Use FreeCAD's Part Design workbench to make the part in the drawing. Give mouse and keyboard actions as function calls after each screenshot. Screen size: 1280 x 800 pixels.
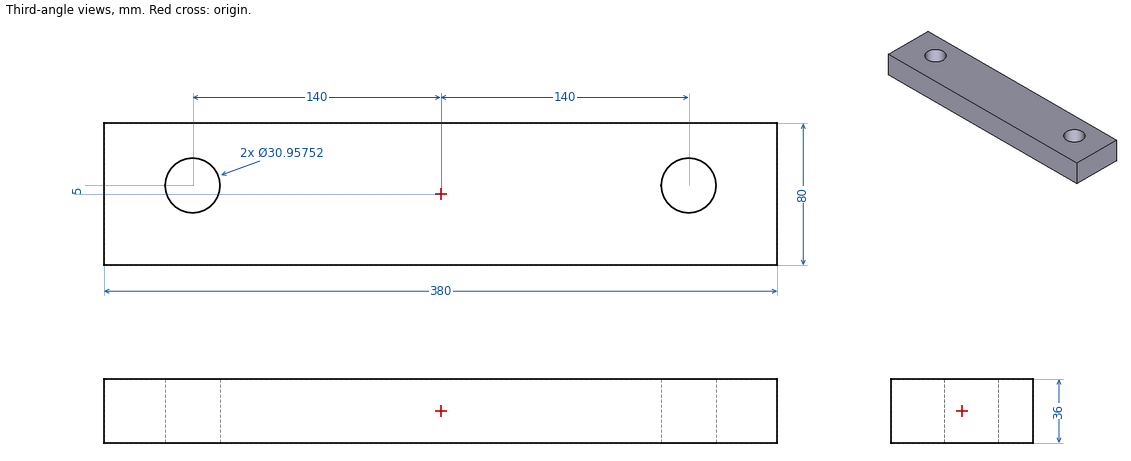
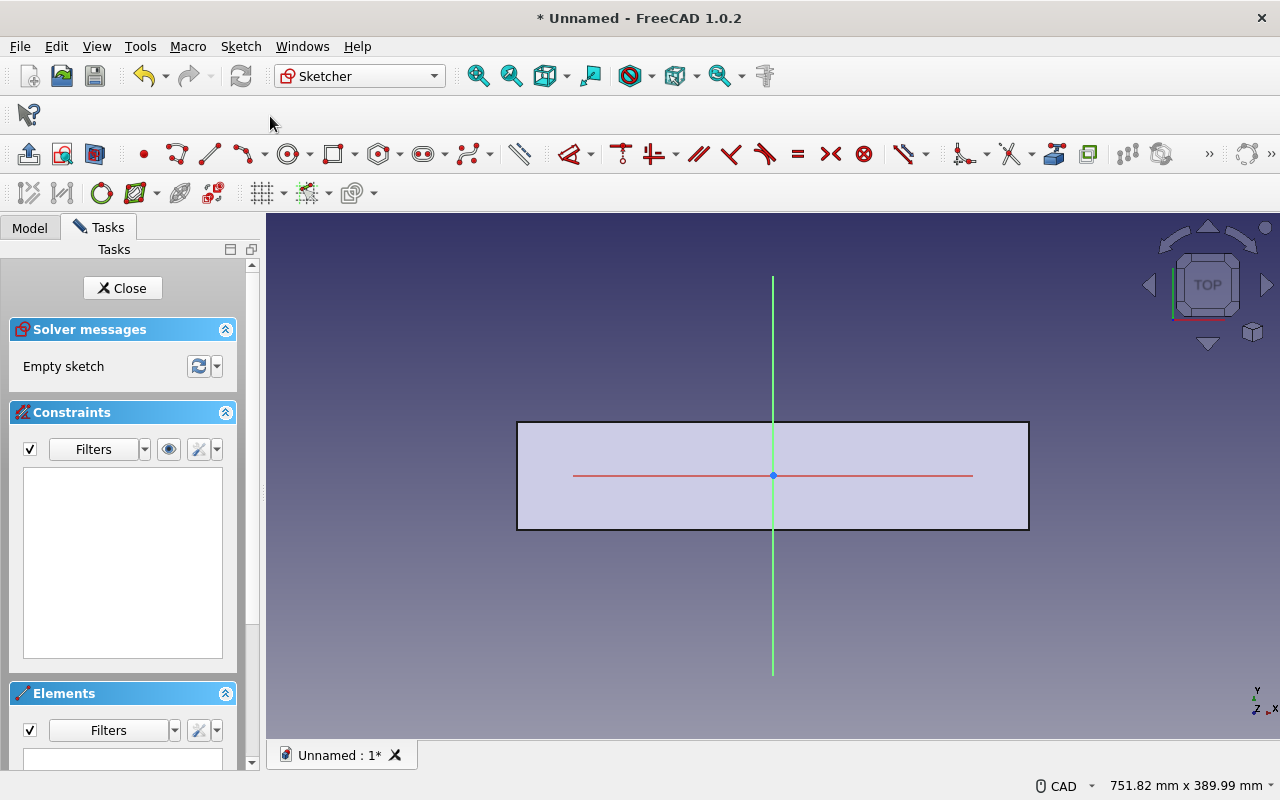
scroll(912, 456, up, 2)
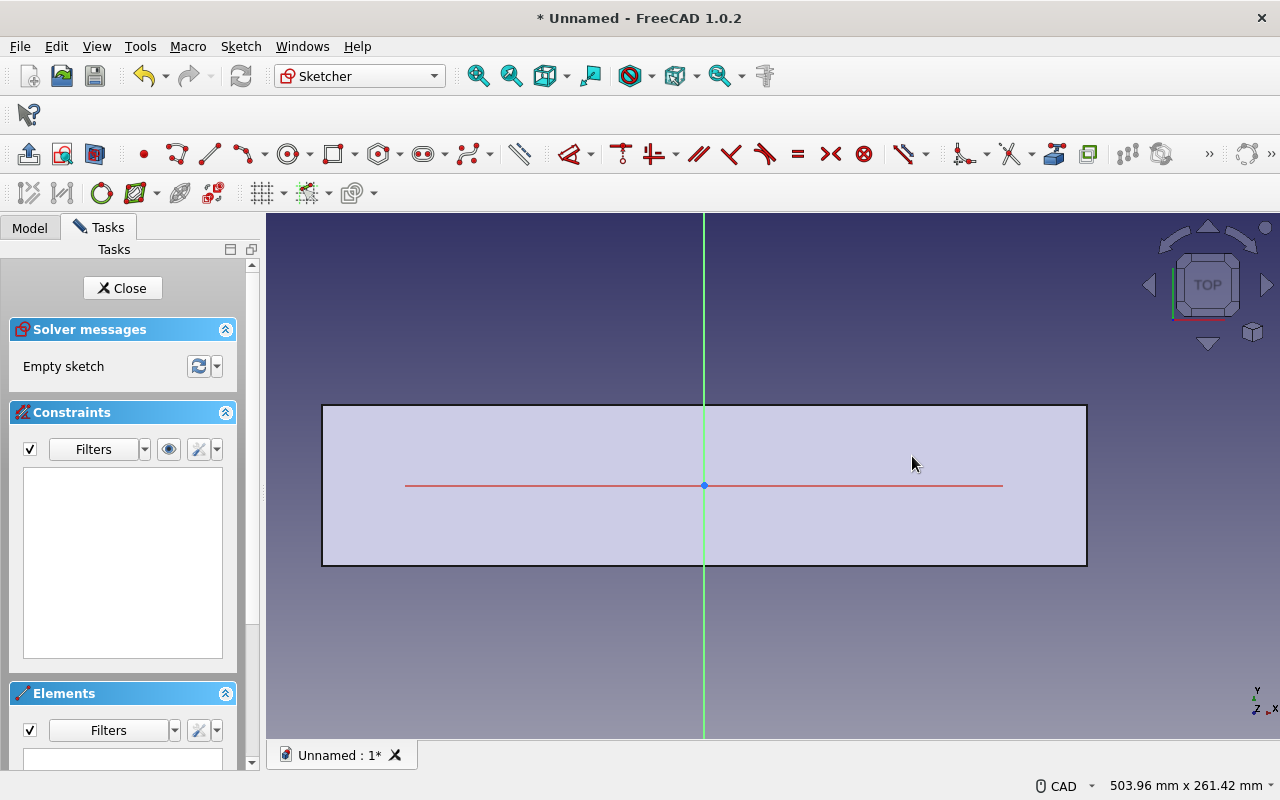
click(288, 154)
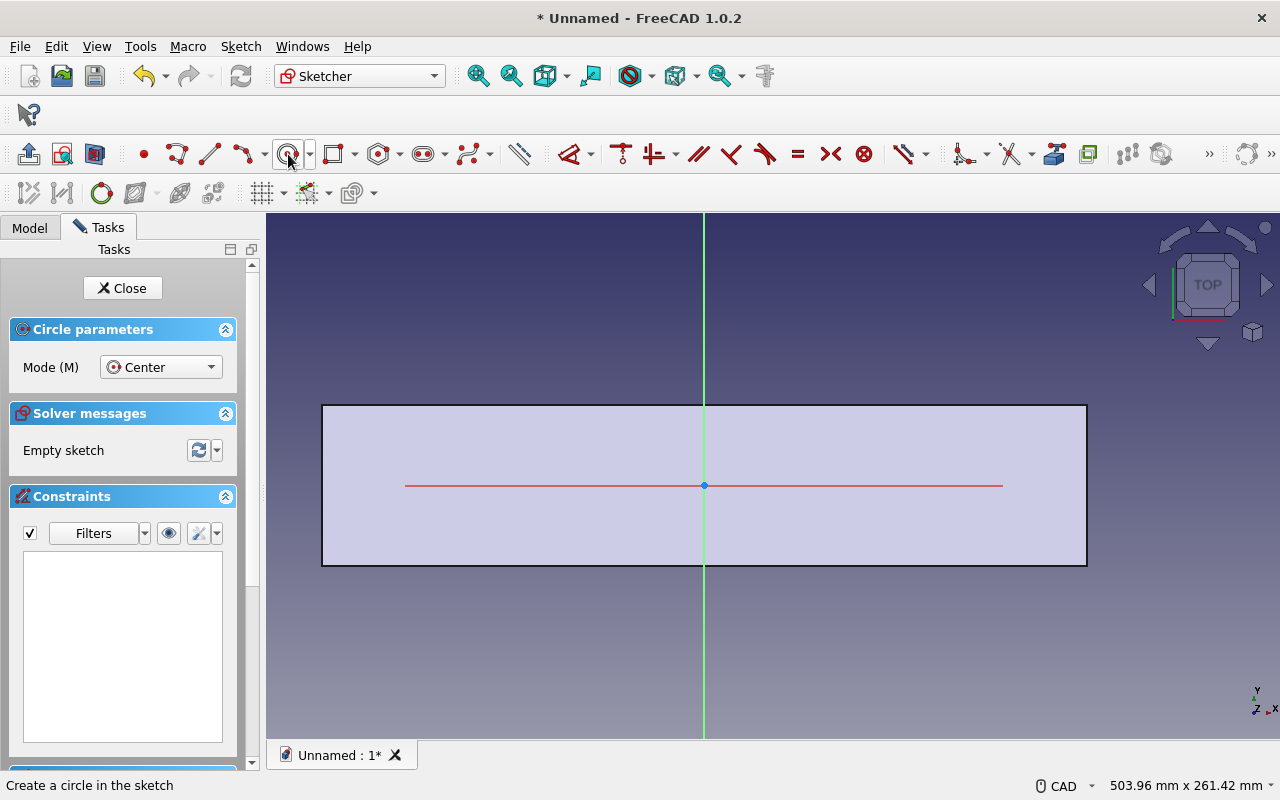
scroll(423, 476, up, 3)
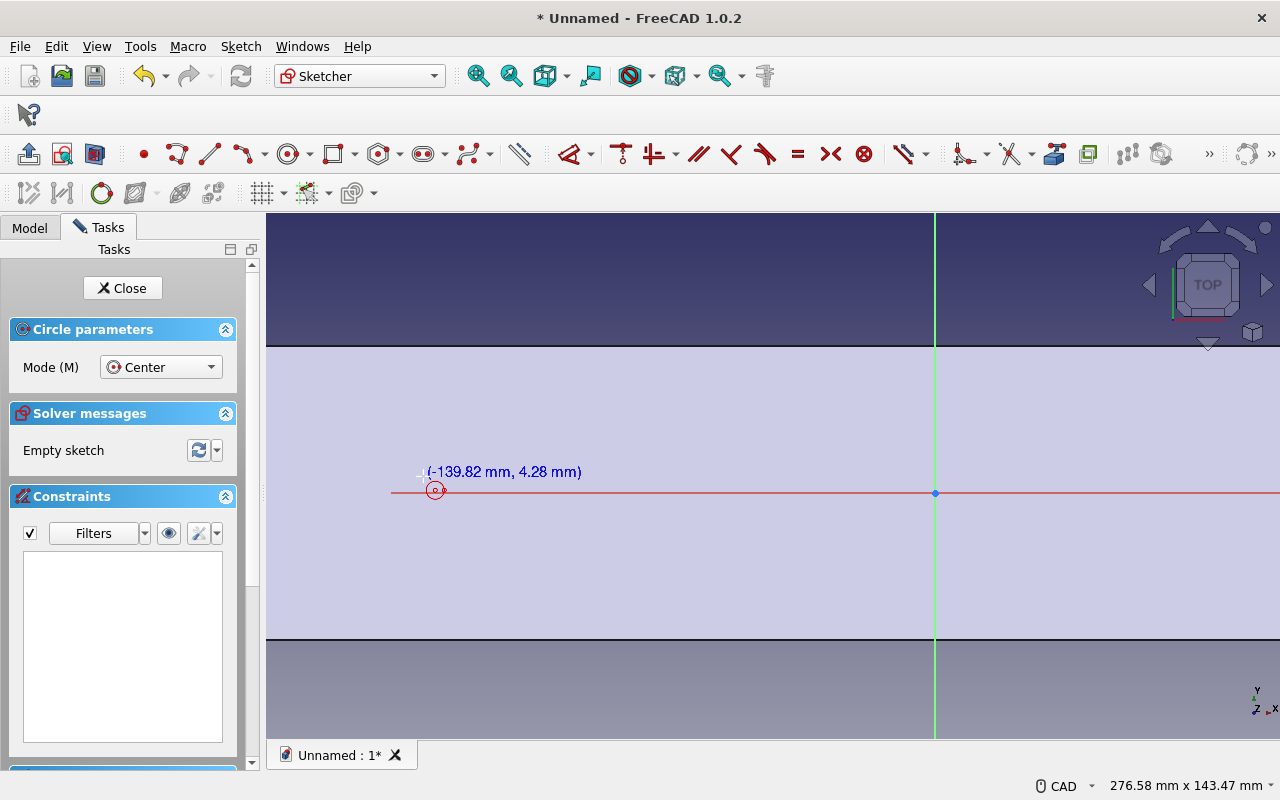
click(422, 475)
click(462, 435)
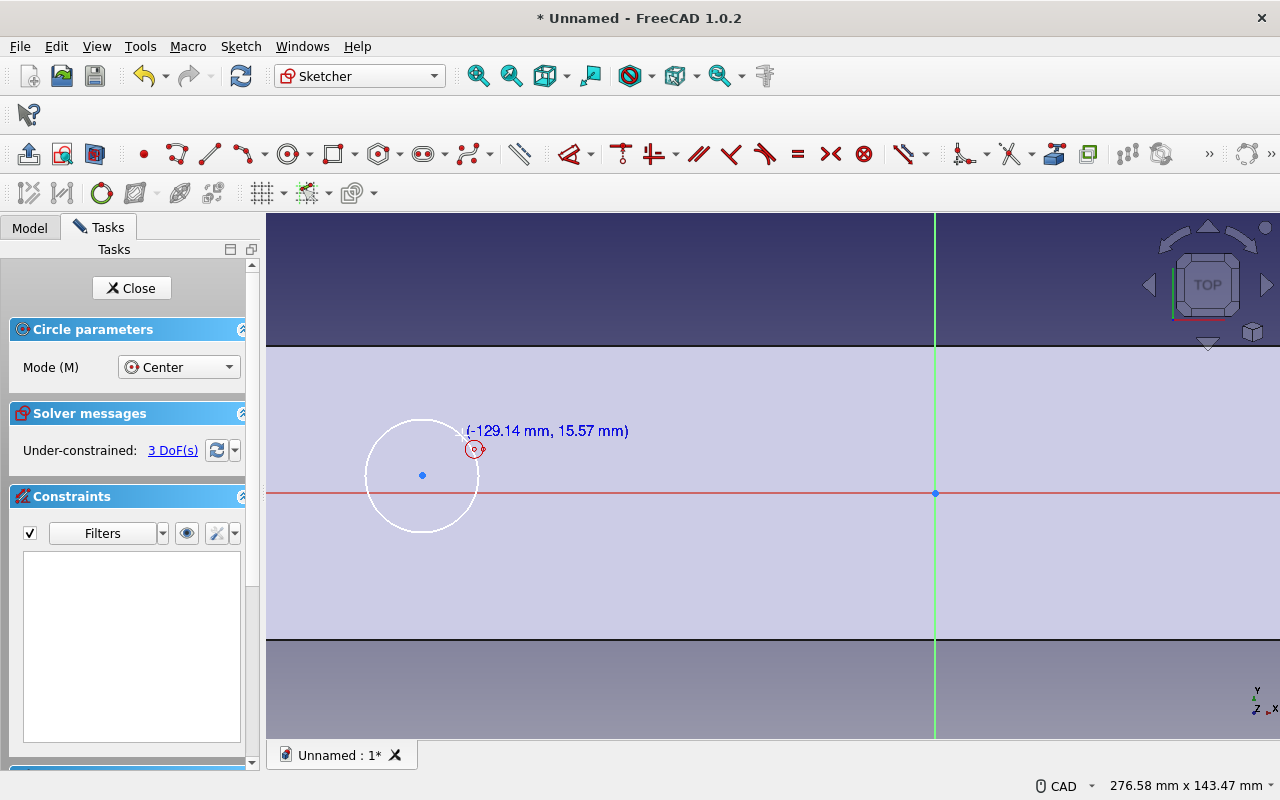
scroll(424, 478, down, 3)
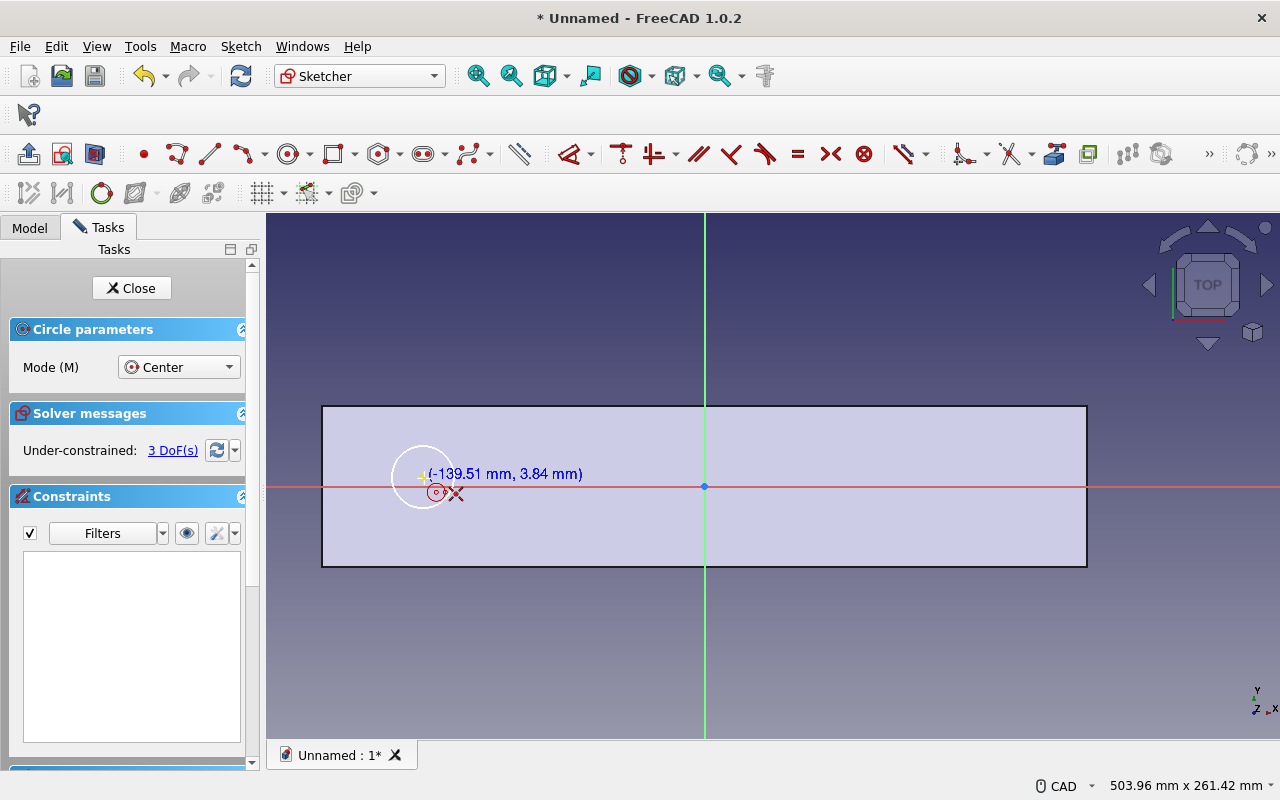
scroll(986, 476, up, 3)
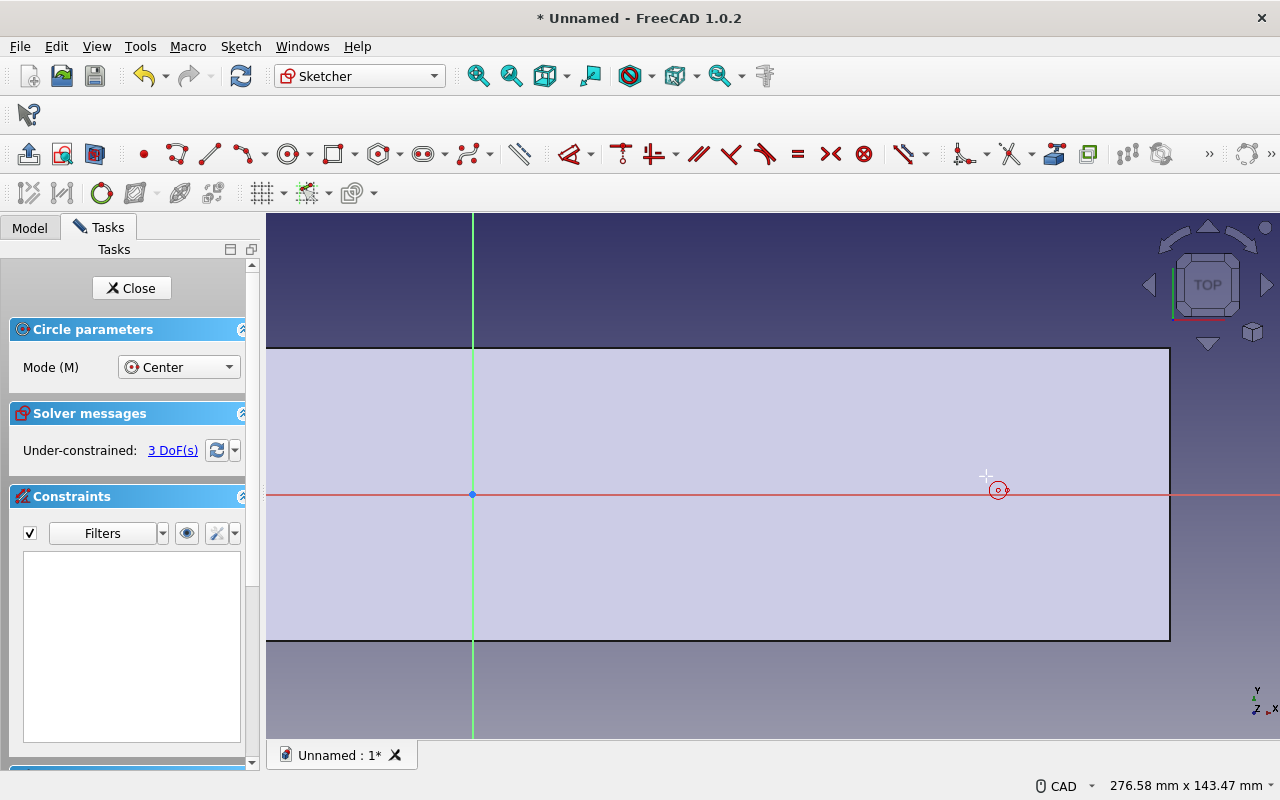
click(986, 476)
click(1026, 436)
key(Escape)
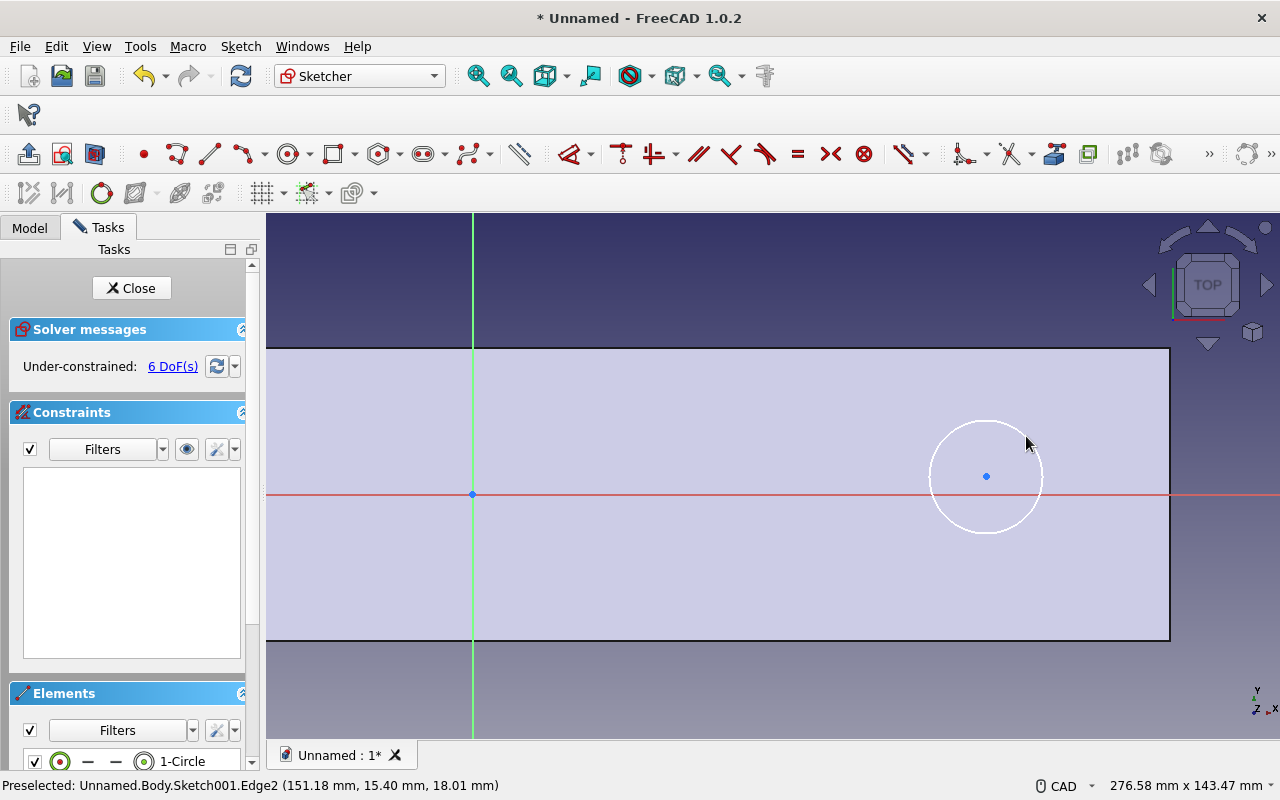
scroll(986, 475, down, 3)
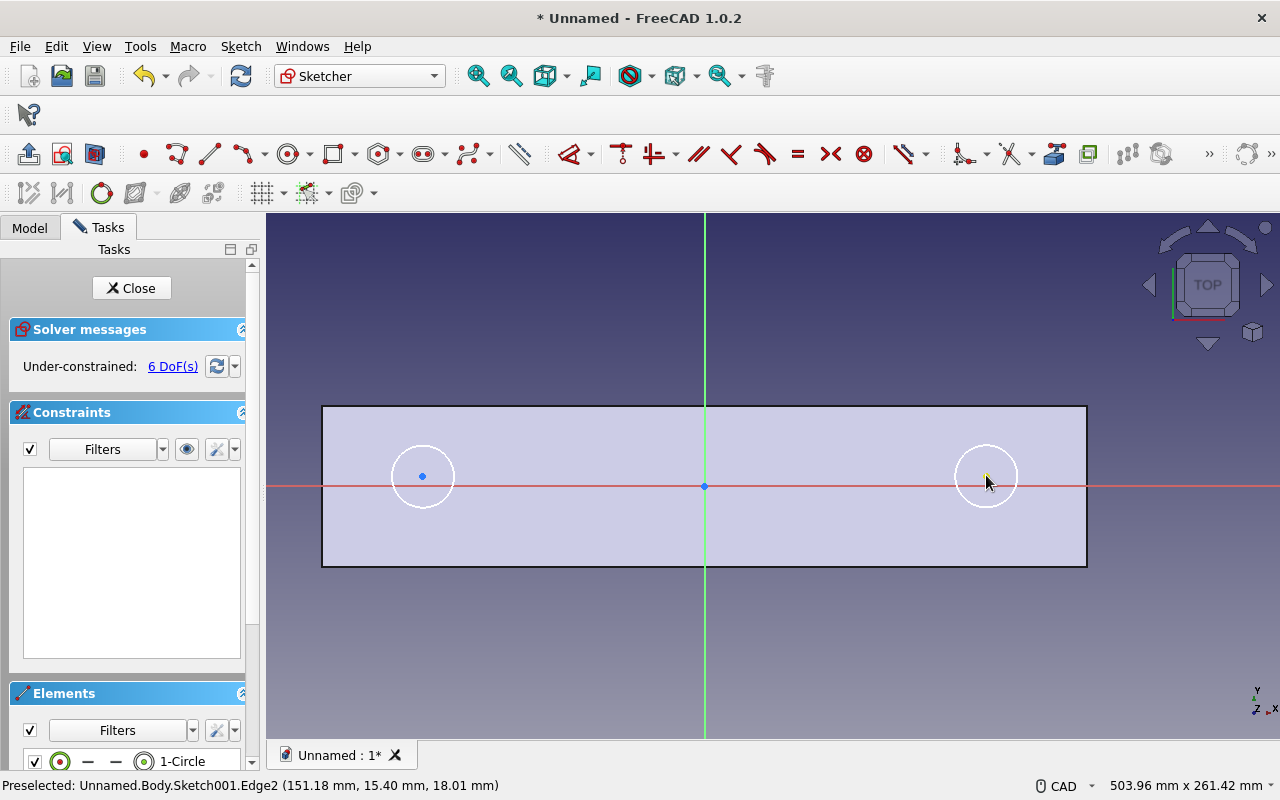
click(445, 455)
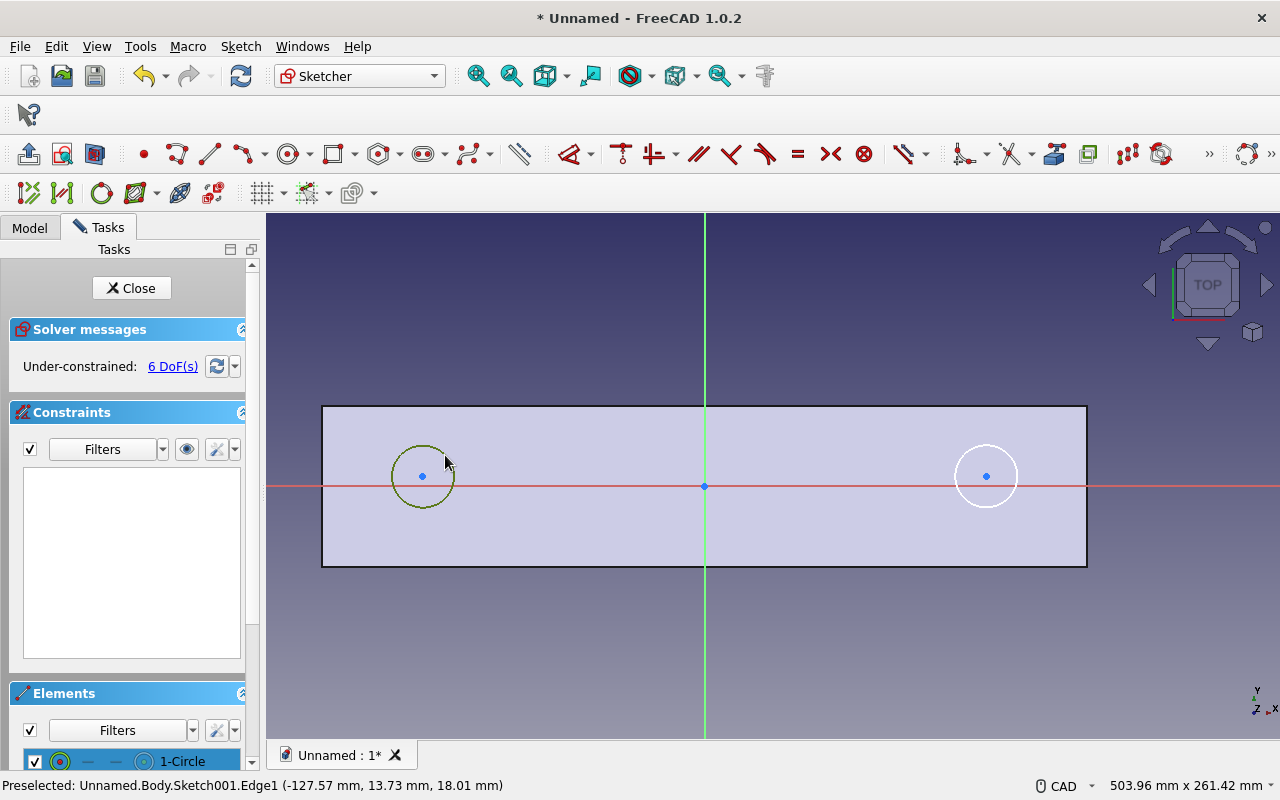
click(1008, 454)